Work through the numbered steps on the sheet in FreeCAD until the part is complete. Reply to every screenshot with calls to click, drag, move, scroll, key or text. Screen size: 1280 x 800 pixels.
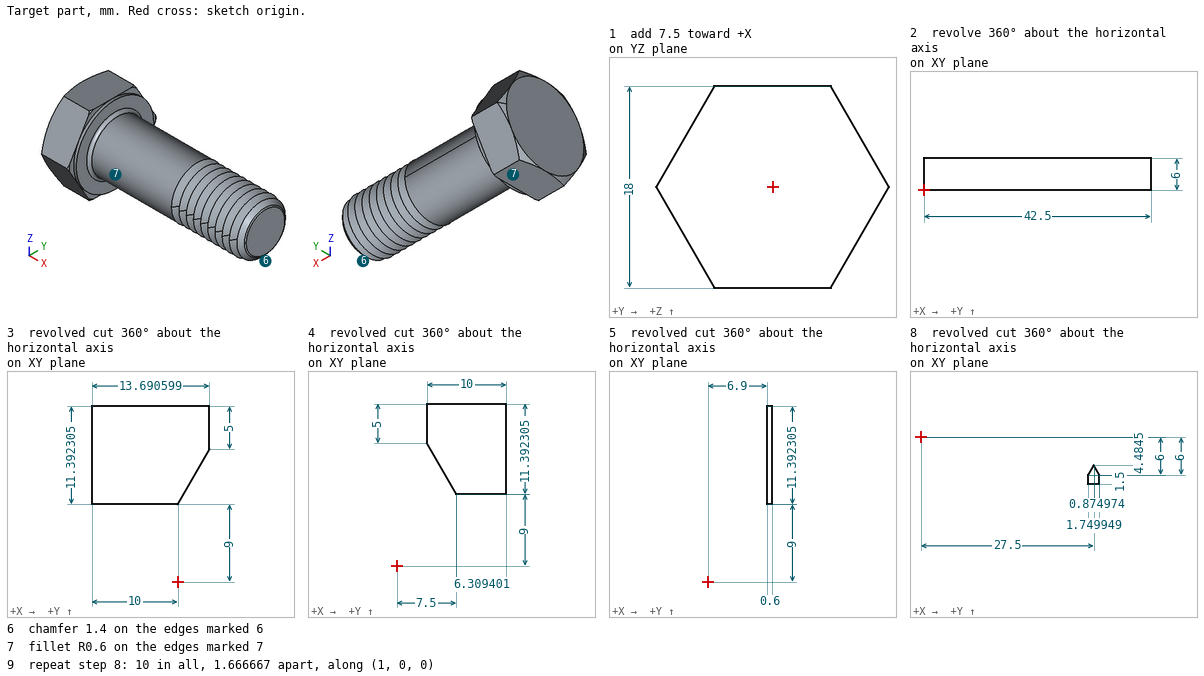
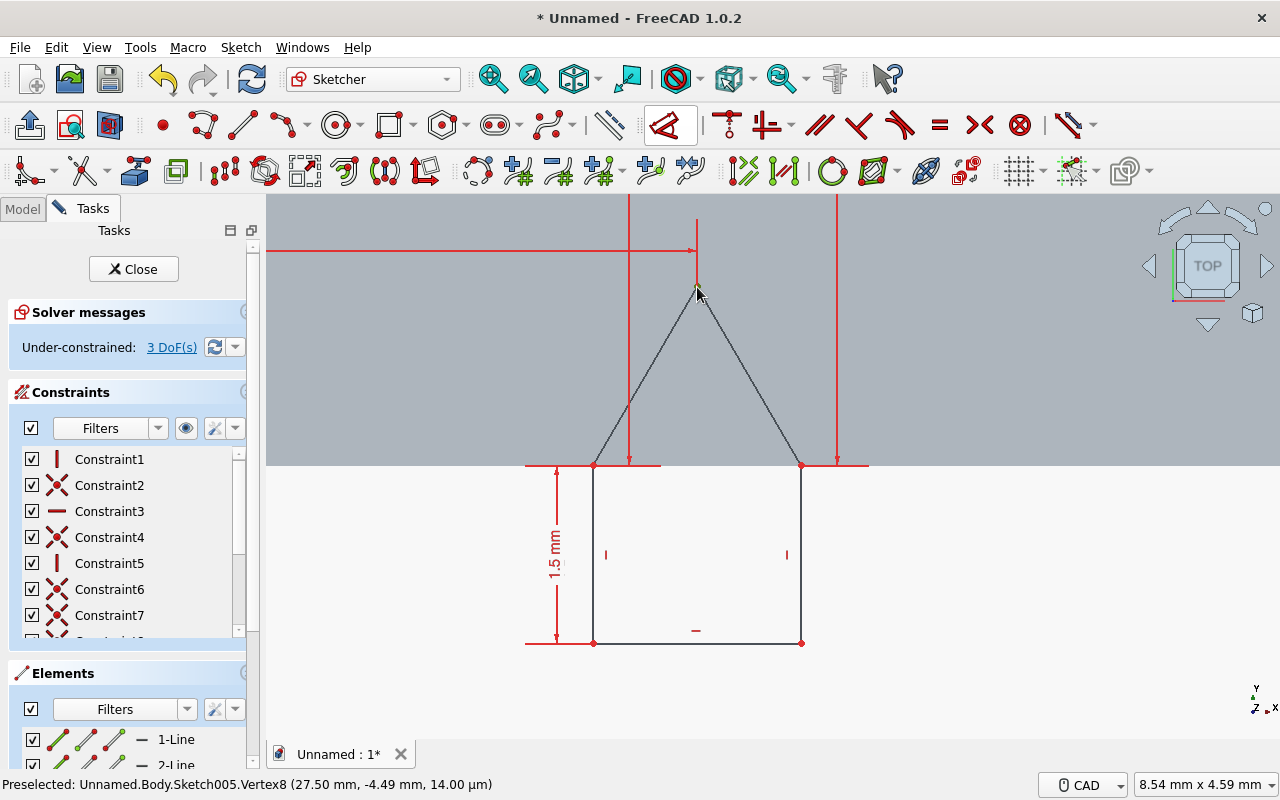
key(i)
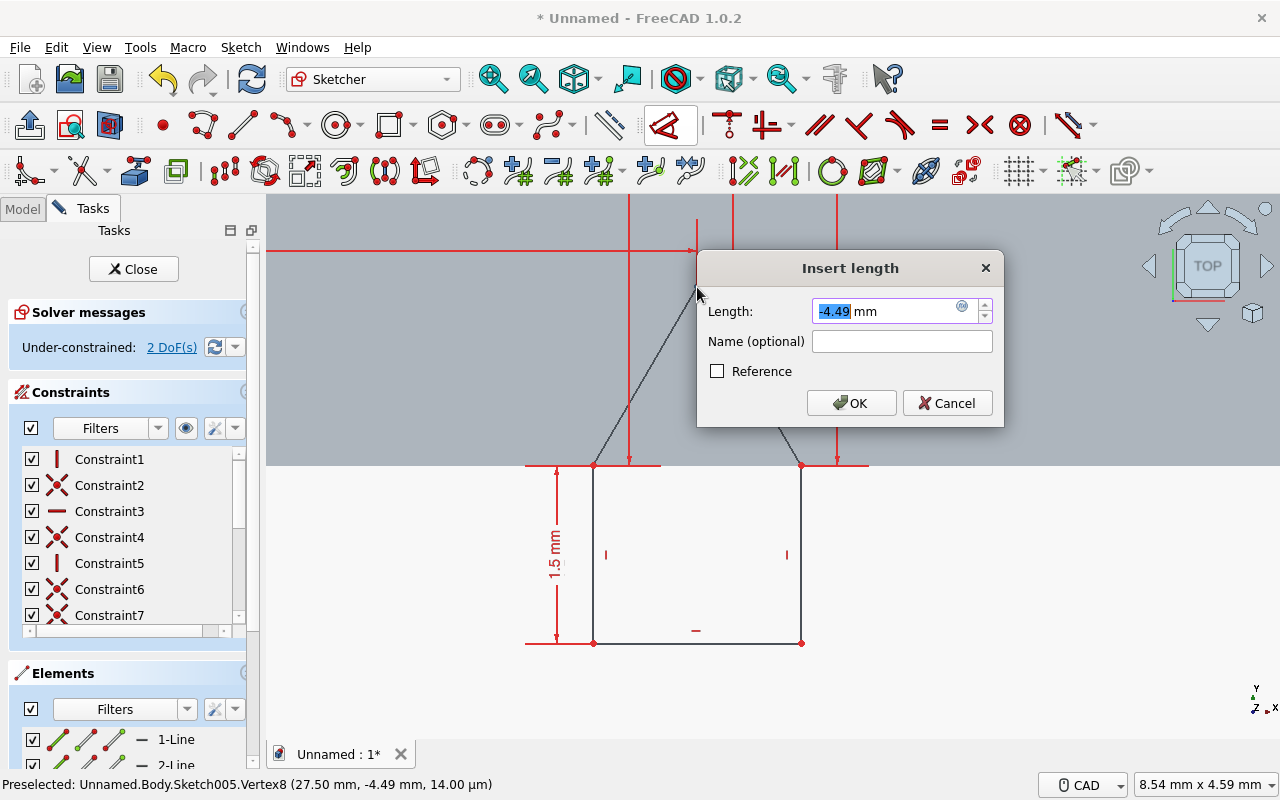
text(-4.4845)
key(Return)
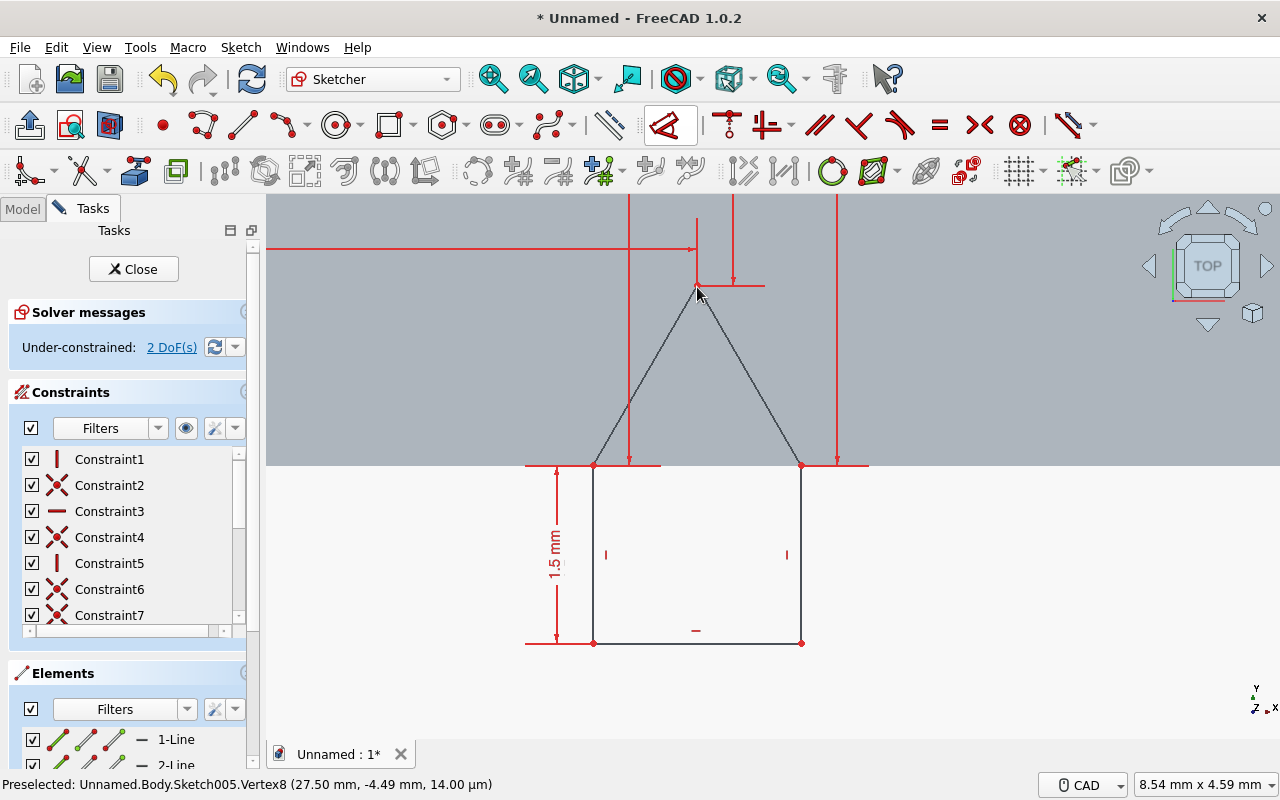
click(655, 644)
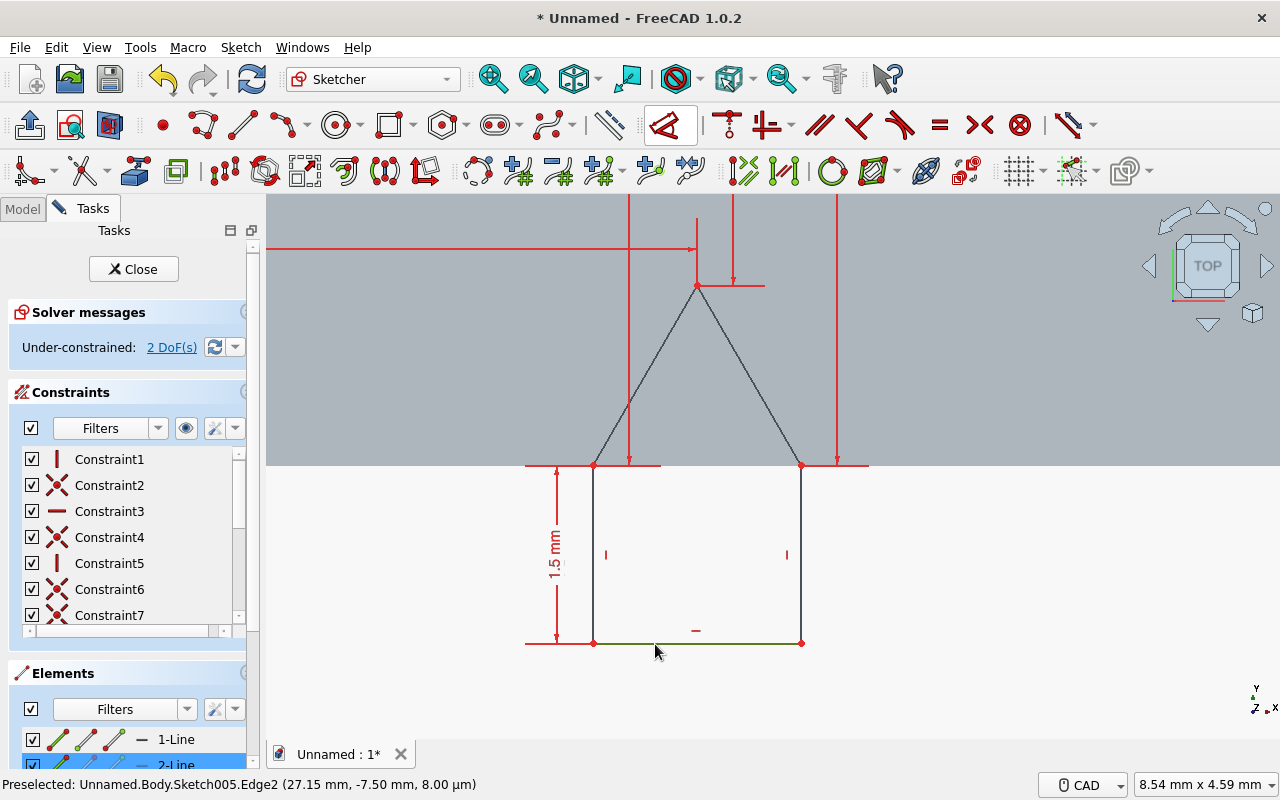
key(l)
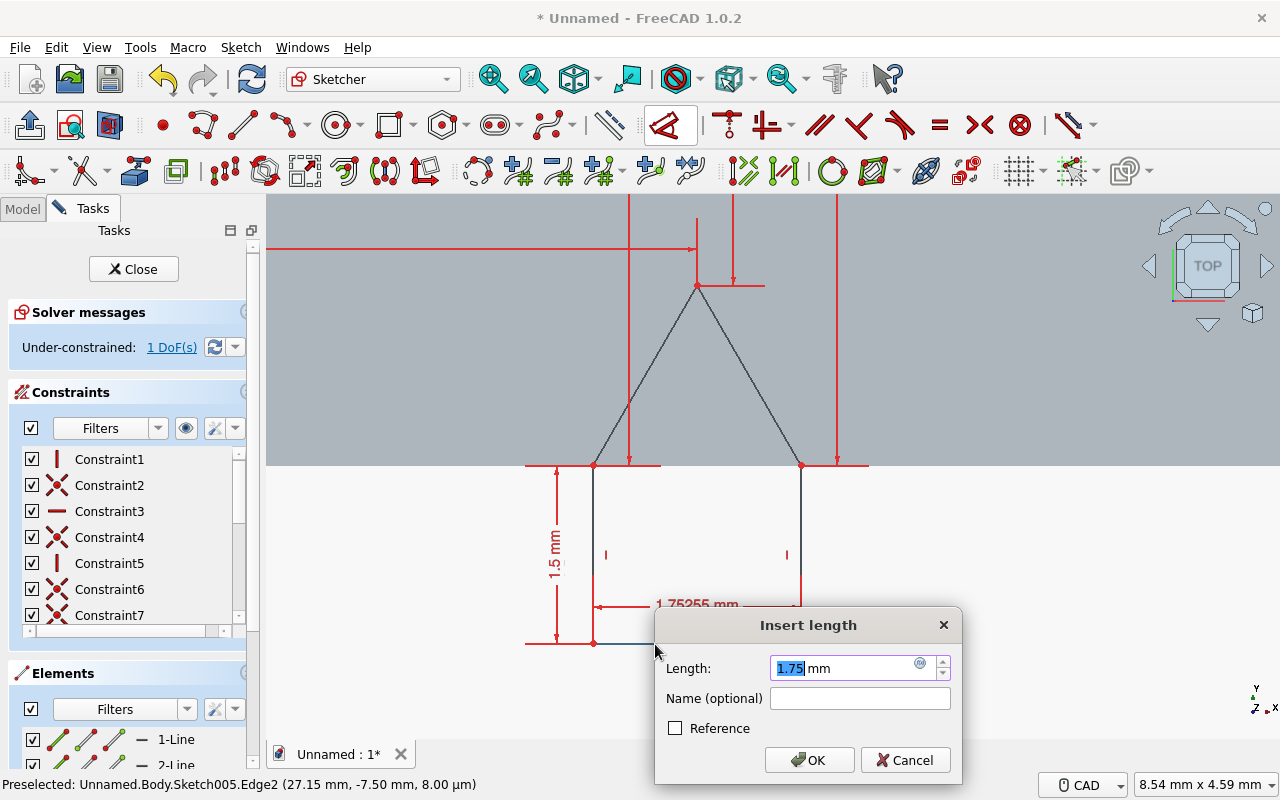
text(1.749949)
key(Return)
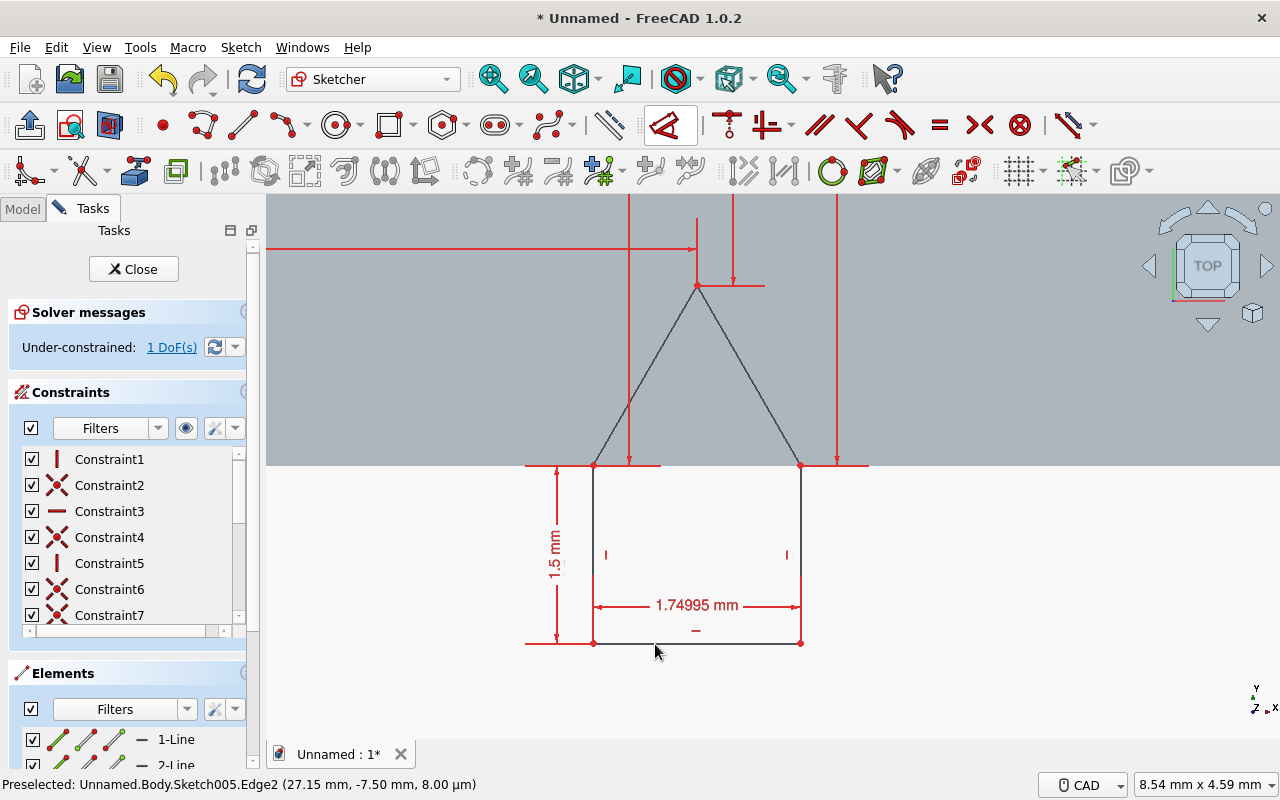
click(770, 412)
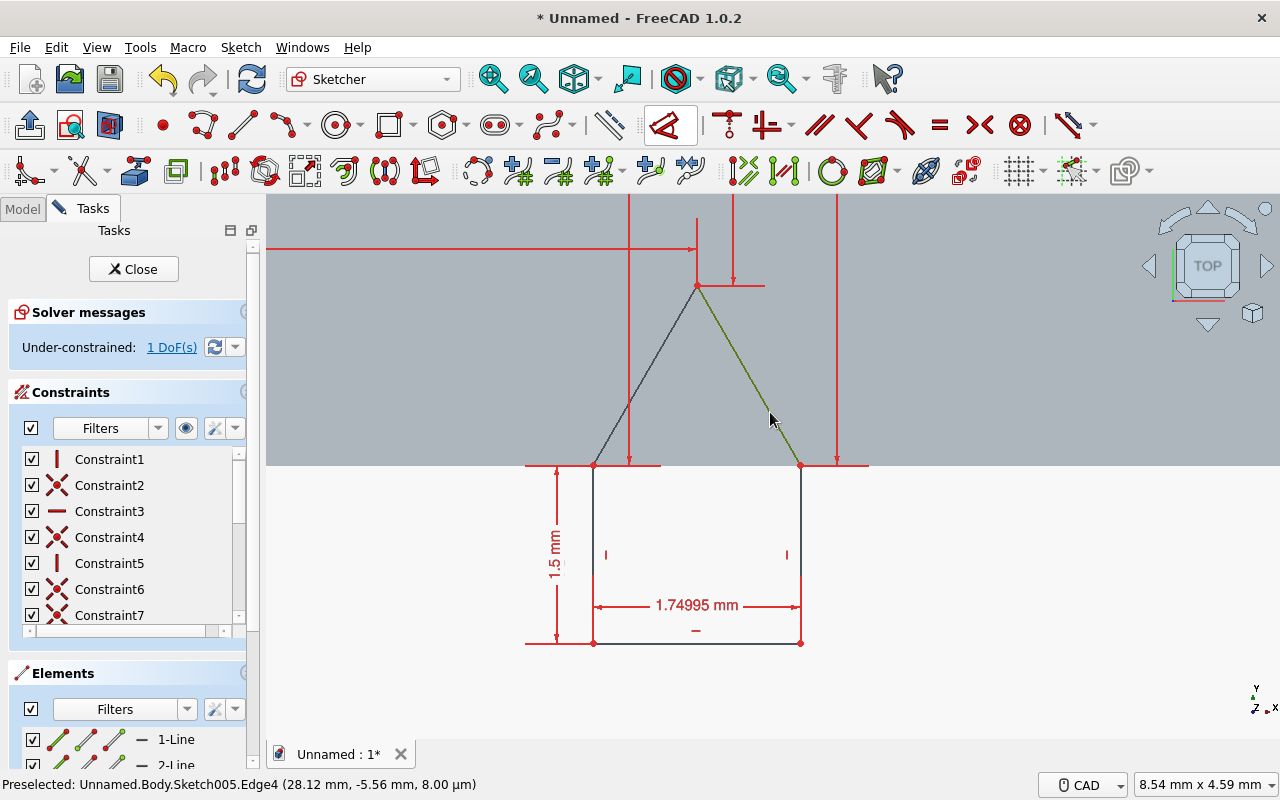
key(l)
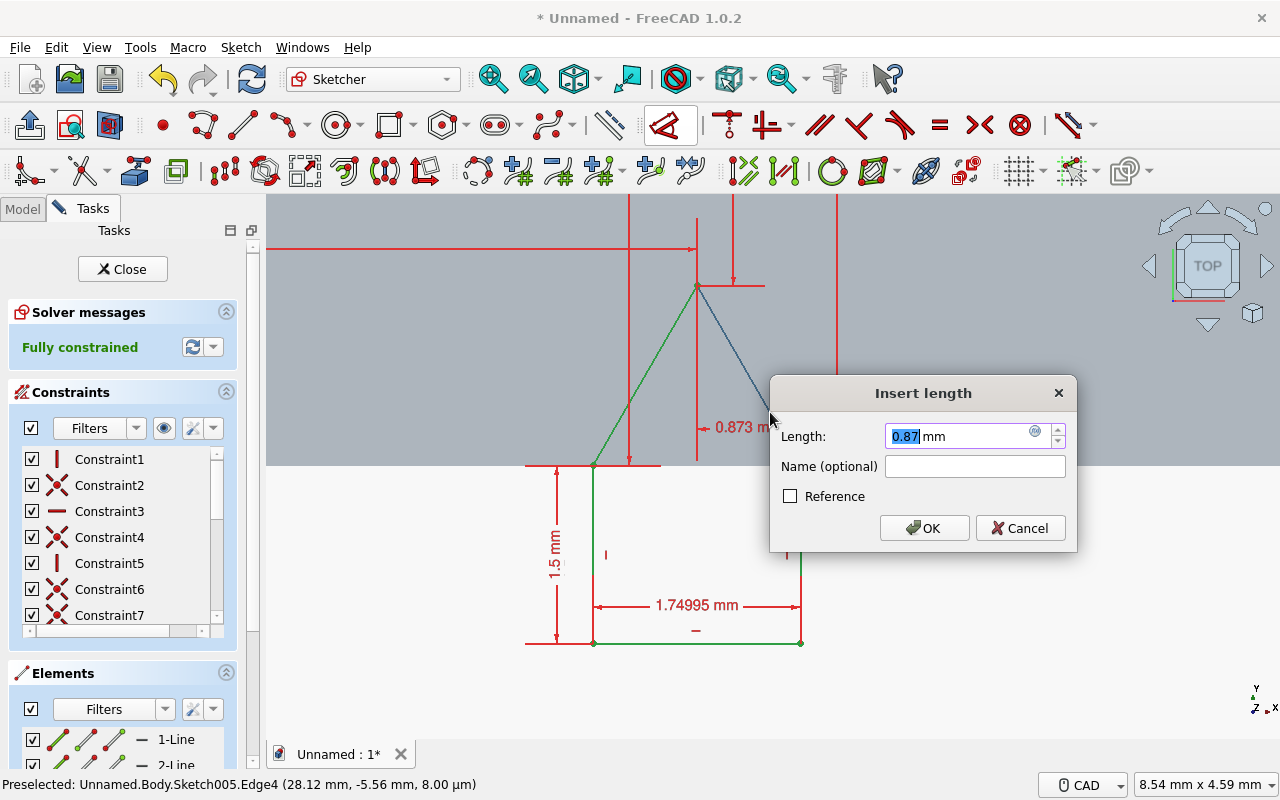
text(0.874974)
key(Return)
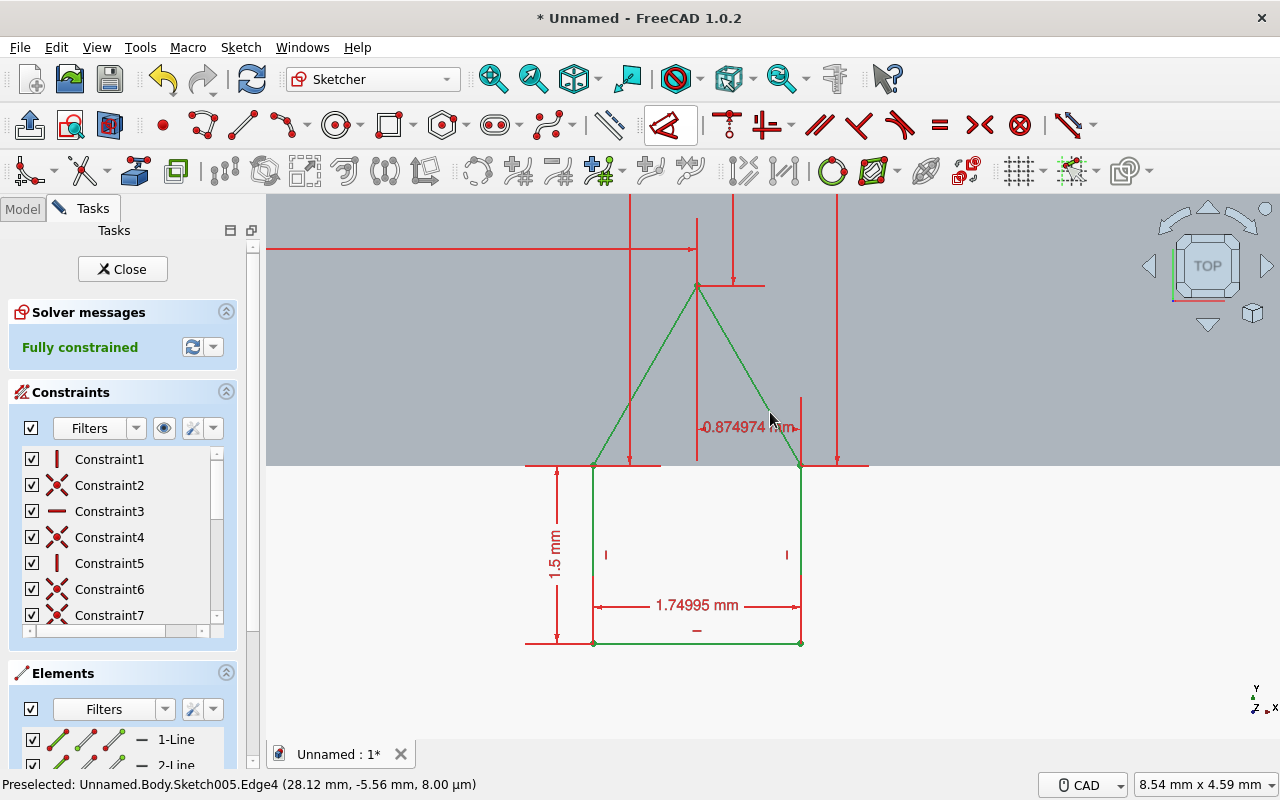
click(123, 269)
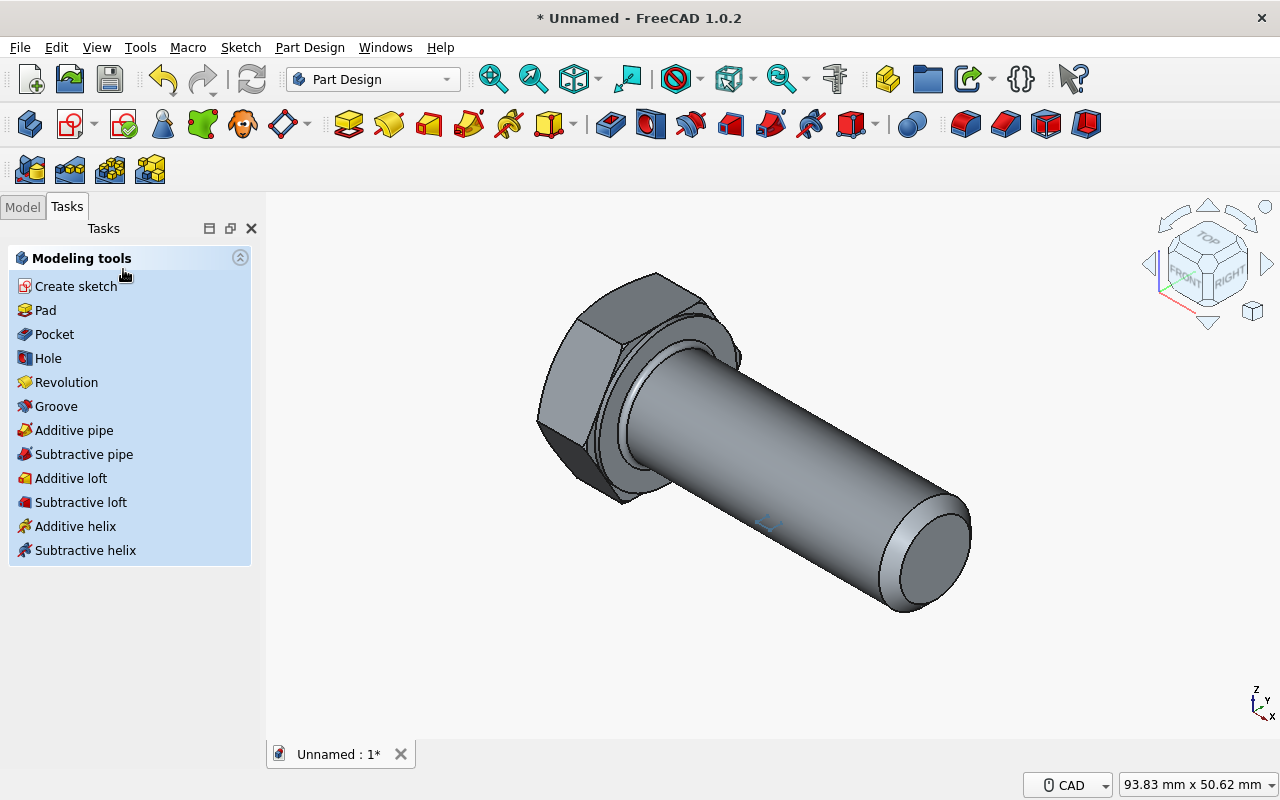
click(692, 124)